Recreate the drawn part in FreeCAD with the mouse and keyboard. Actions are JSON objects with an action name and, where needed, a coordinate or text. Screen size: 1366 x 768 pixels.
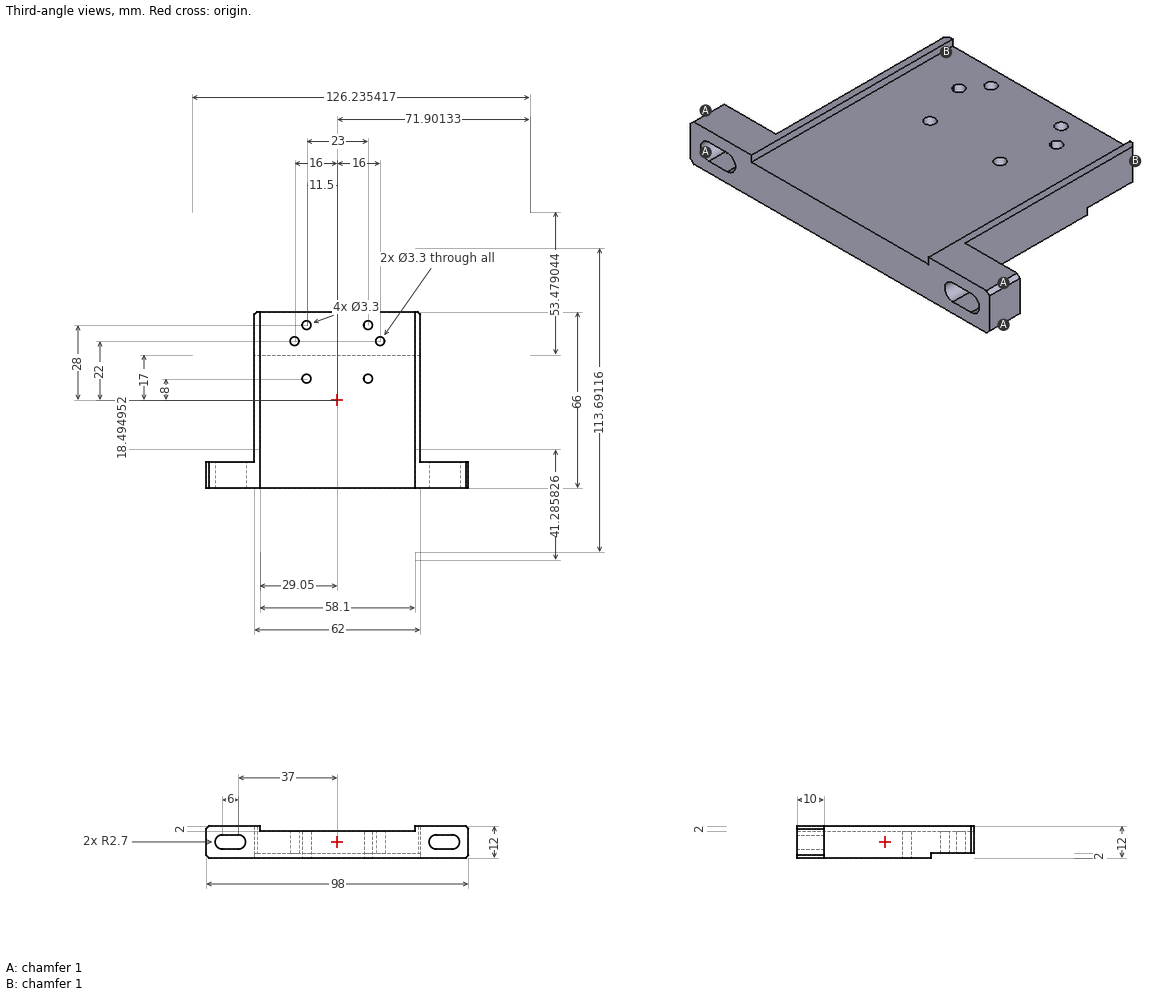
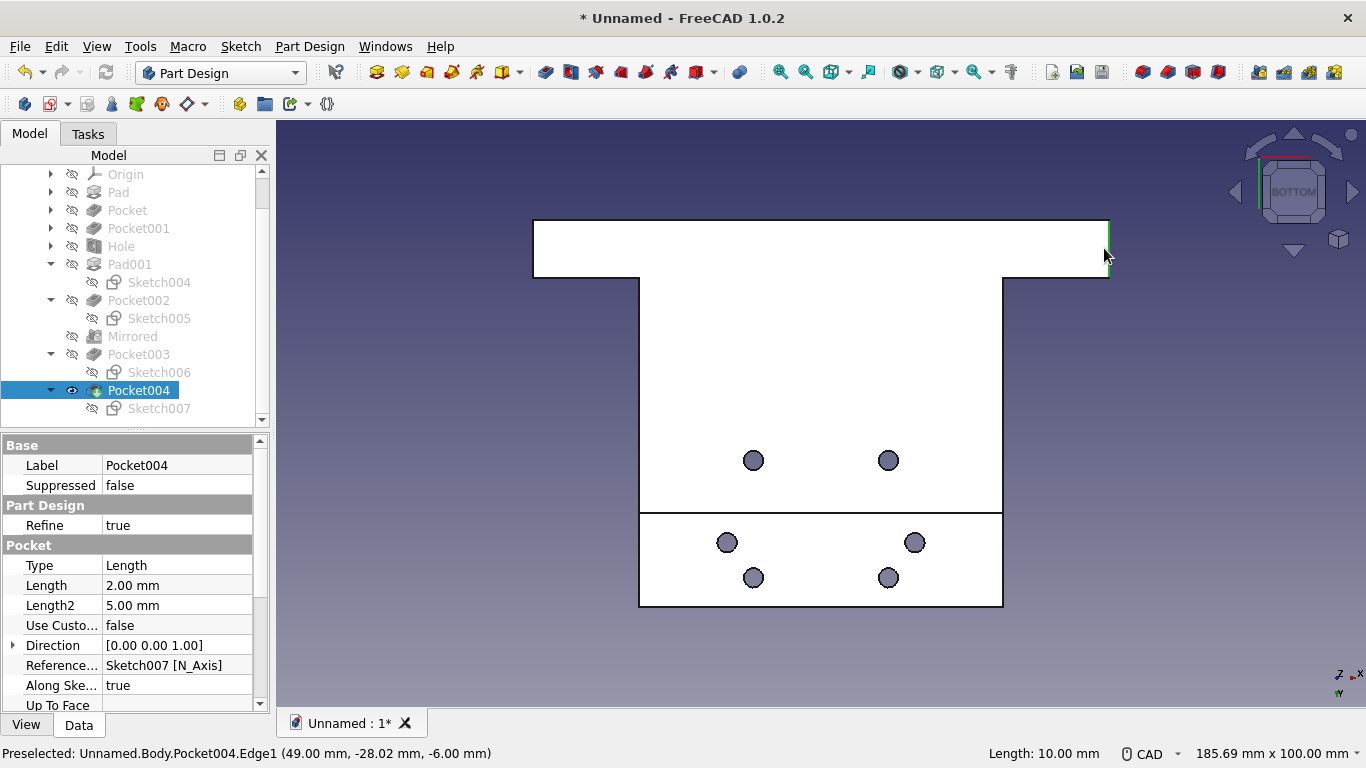
{"action": "left_click", "coordinate": [533, 248], "text": "ctrl"}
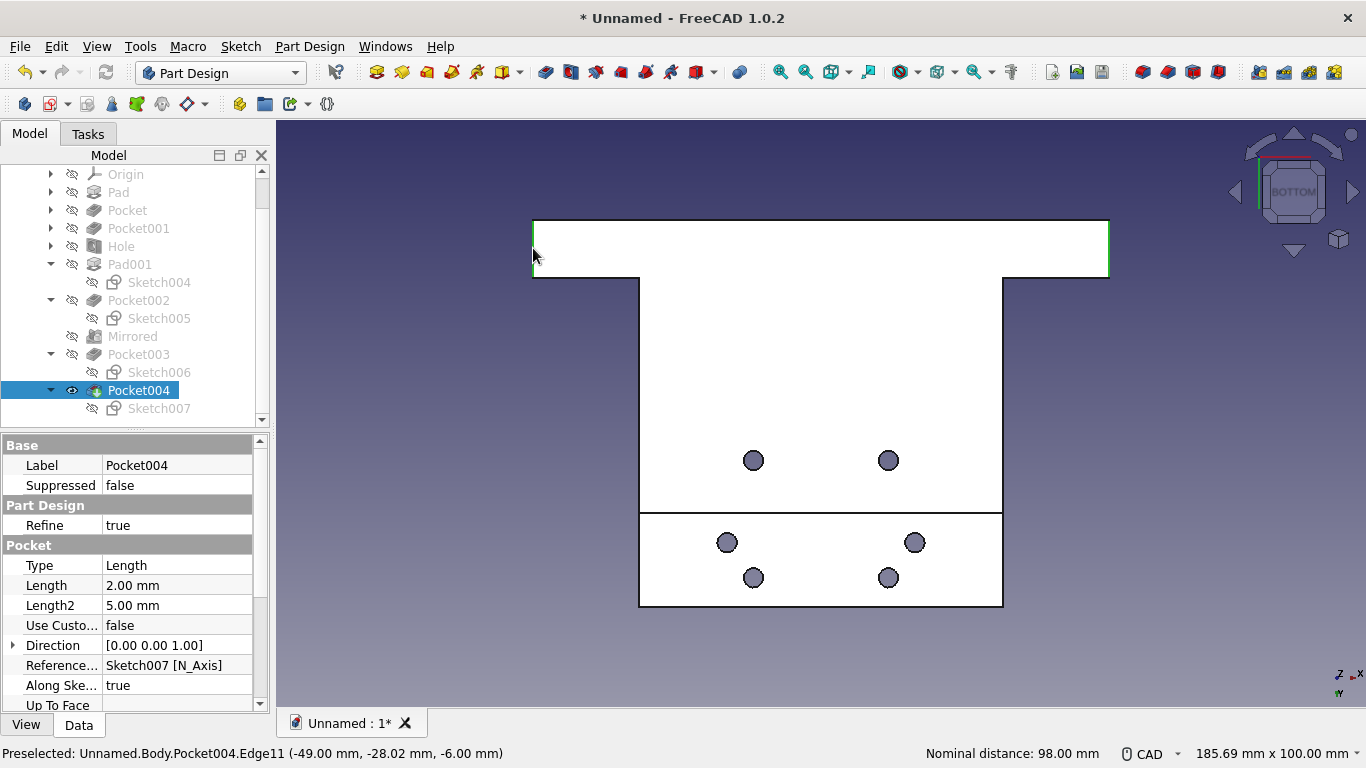
{"action": "key", "text": "0"}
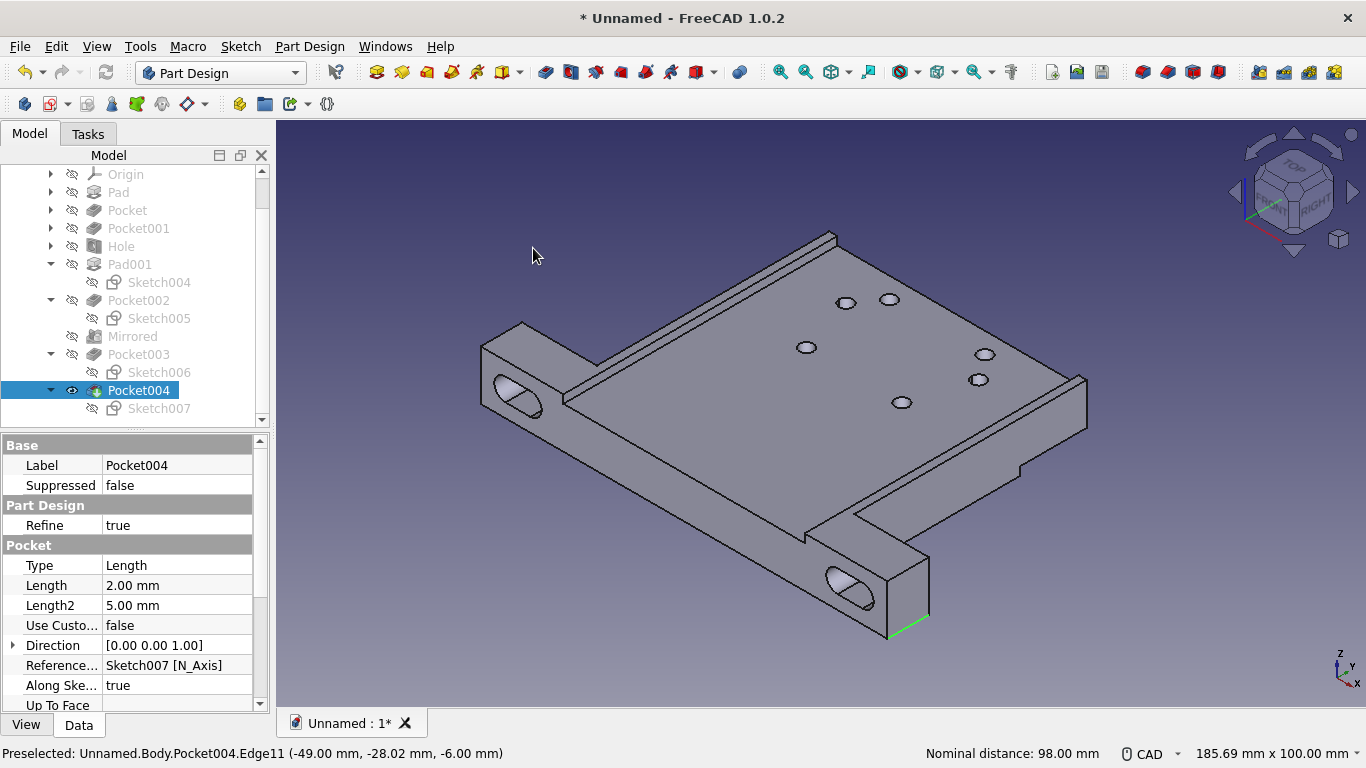
{"action": "left_click", "coordinate": [908, 568], "text": "ctrl"}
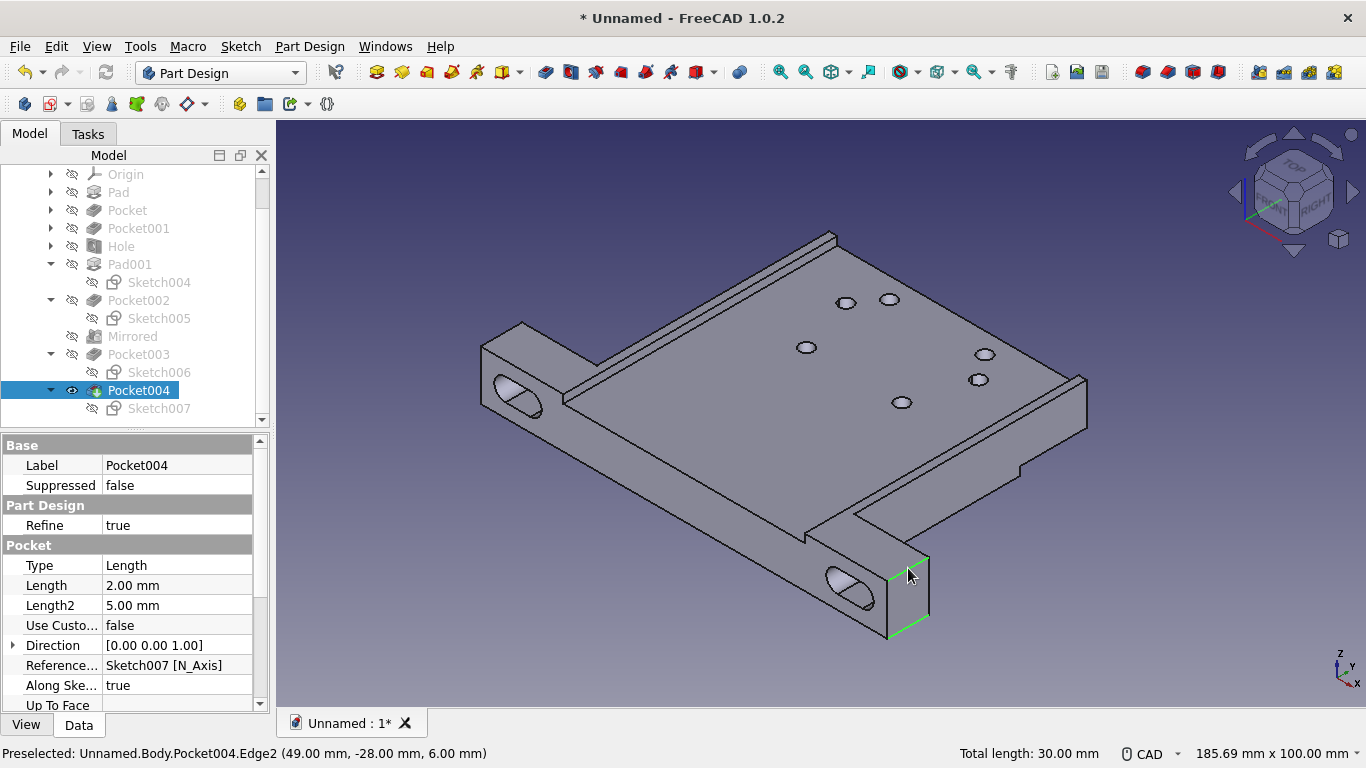
{"action": "key", "text": "2"}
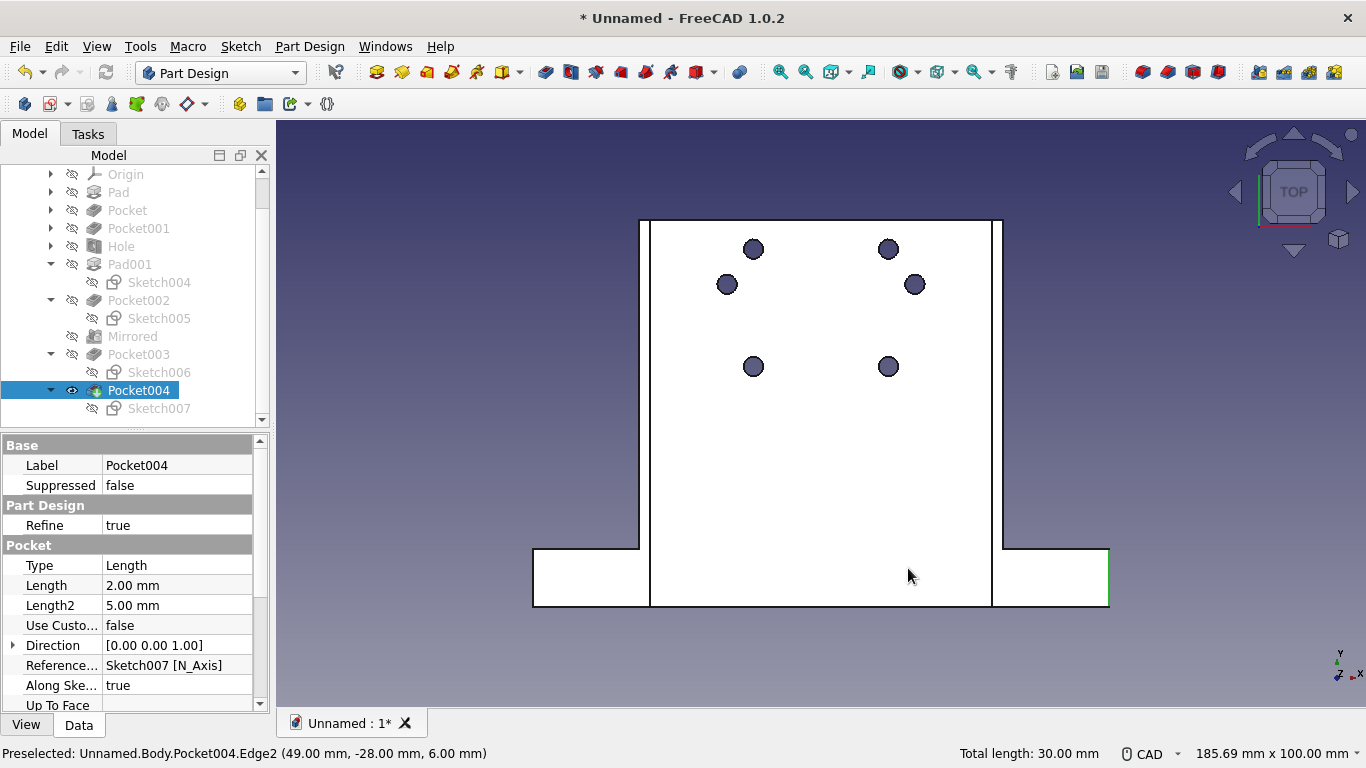
{"action": "left_click", "coordinate": [533, 577], "text": "ctrl"}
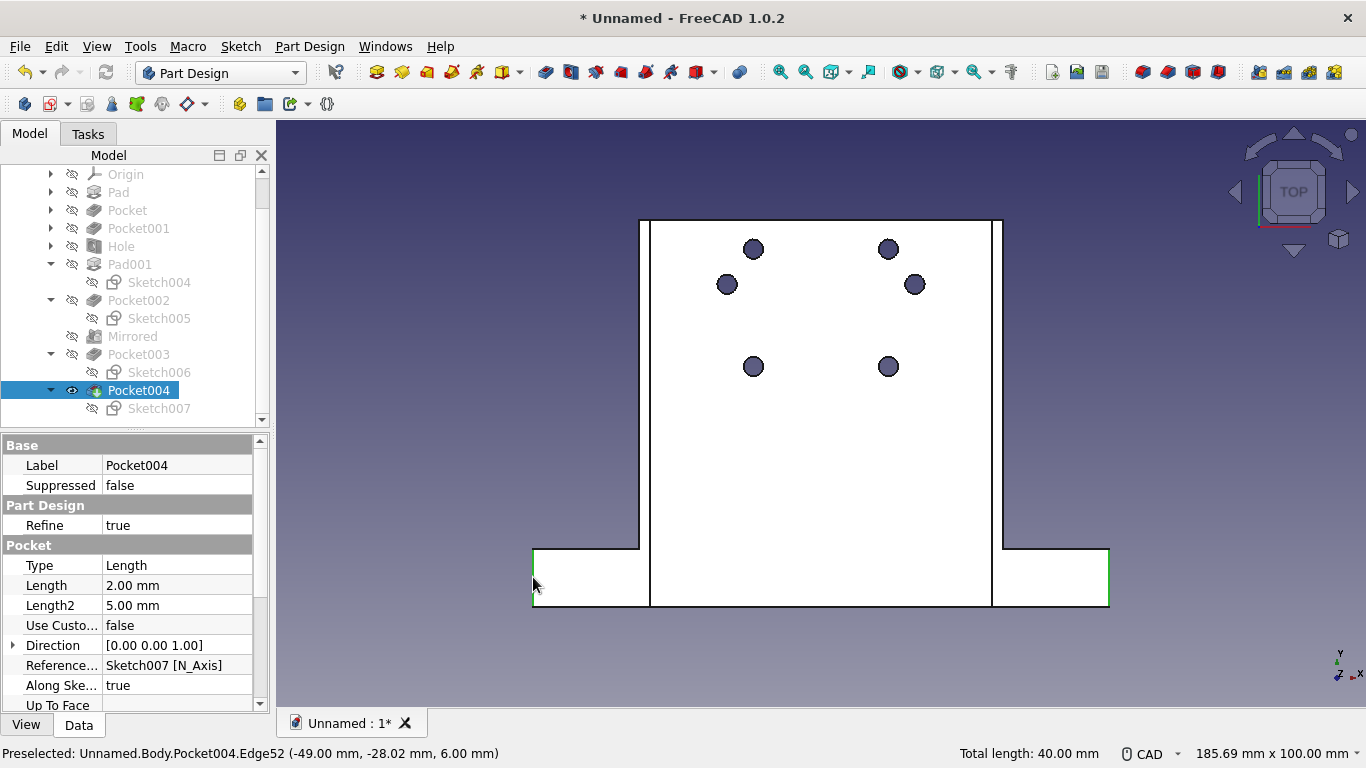
{"action": "left_click", "coordinate": [1168, 72]}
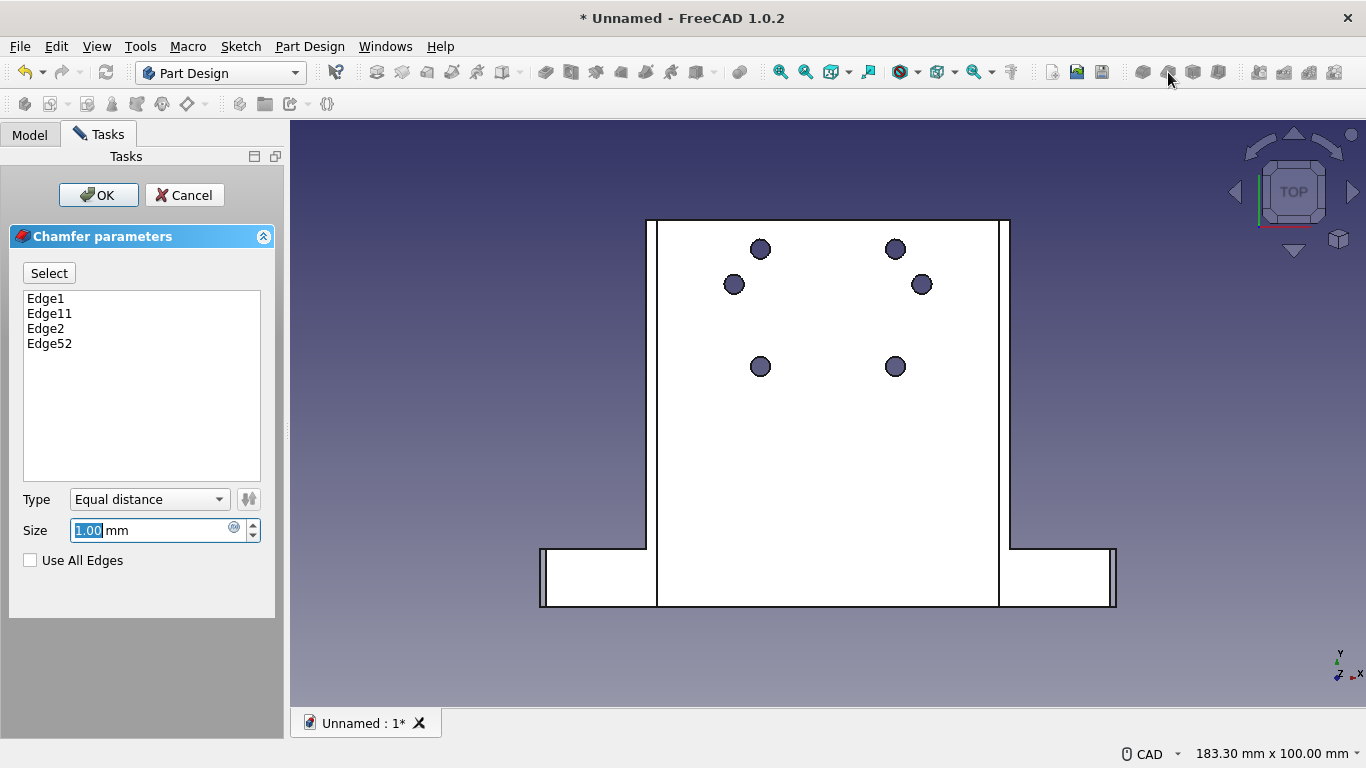
{"action": "type", "text": "1"}
{"action": "key", "text": "Tab"}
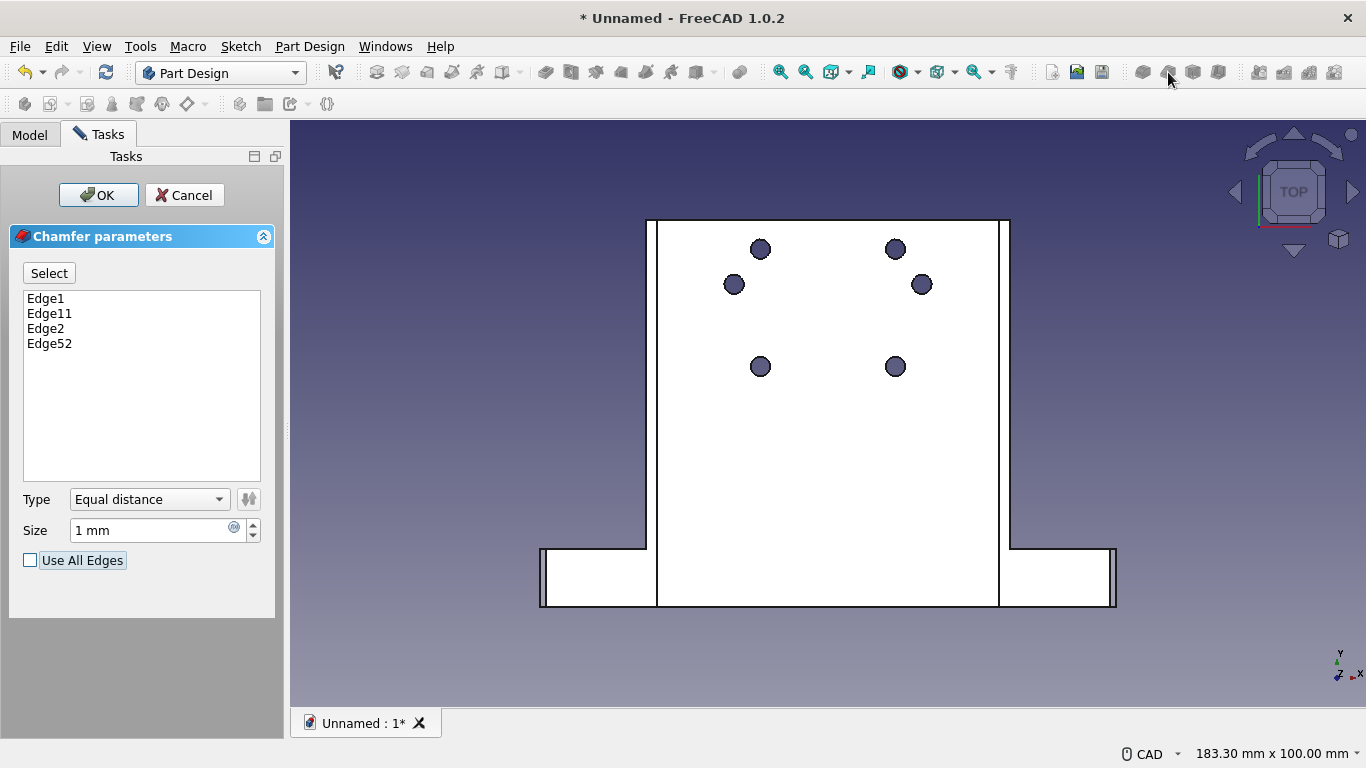
{"action": "left_click", "coordinate": [99, 195]}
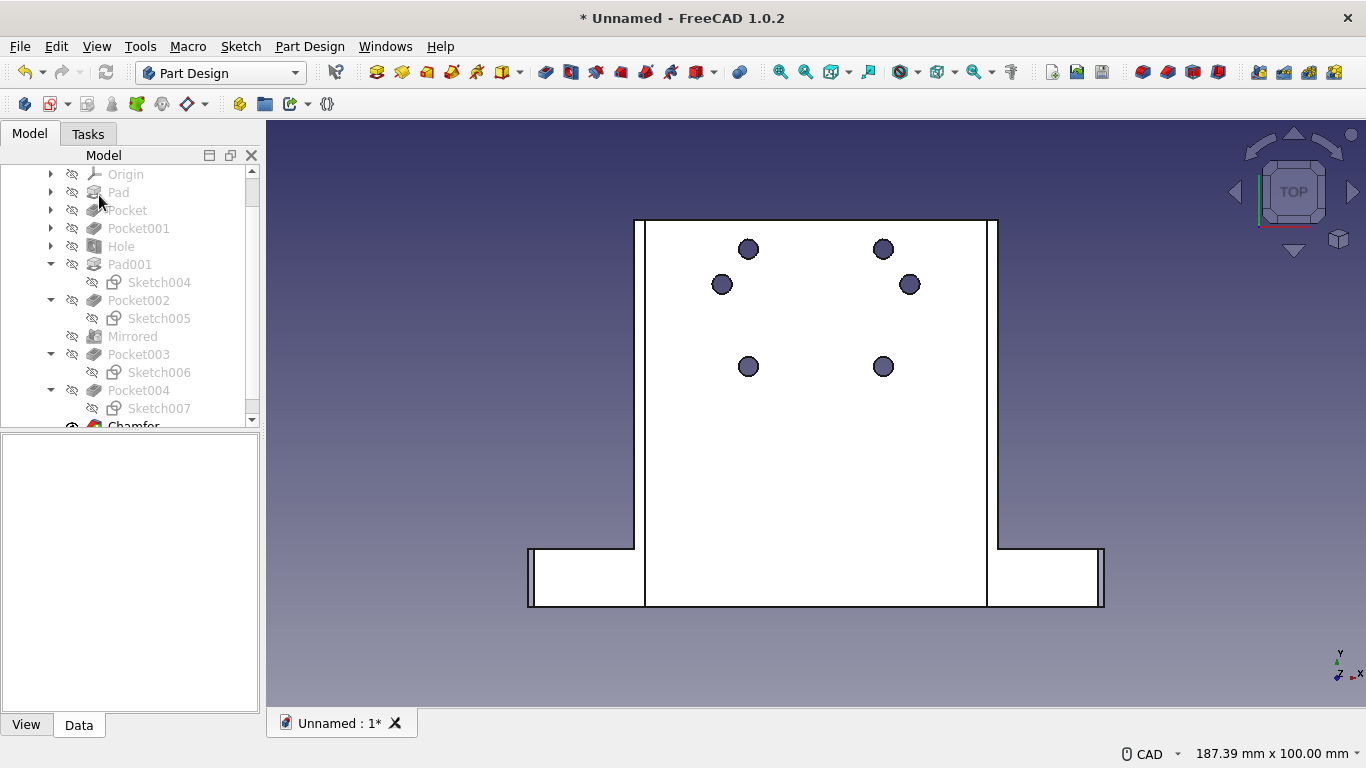
{"action": "key", "text": "0"}